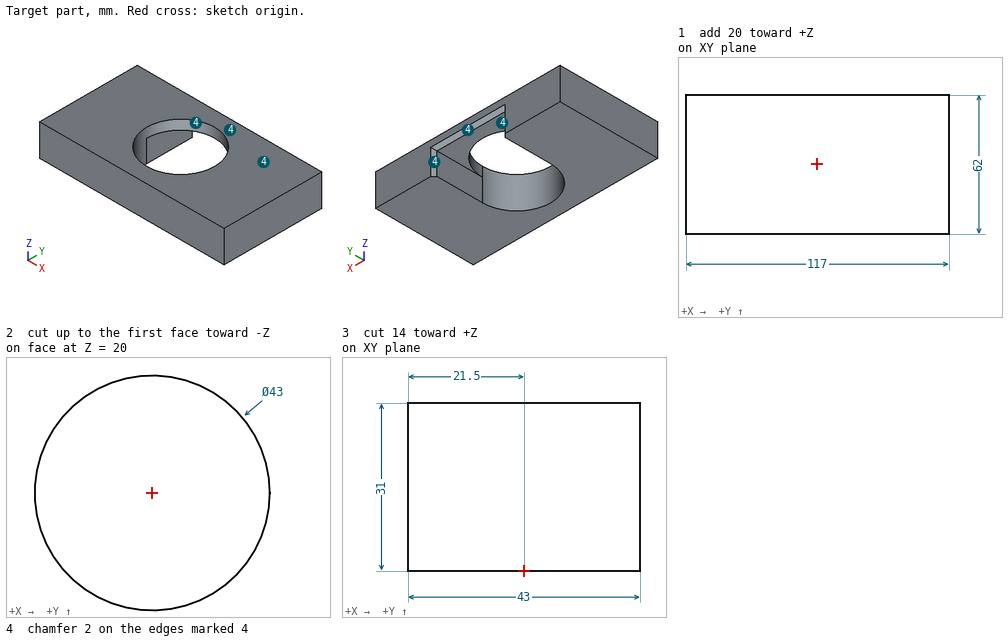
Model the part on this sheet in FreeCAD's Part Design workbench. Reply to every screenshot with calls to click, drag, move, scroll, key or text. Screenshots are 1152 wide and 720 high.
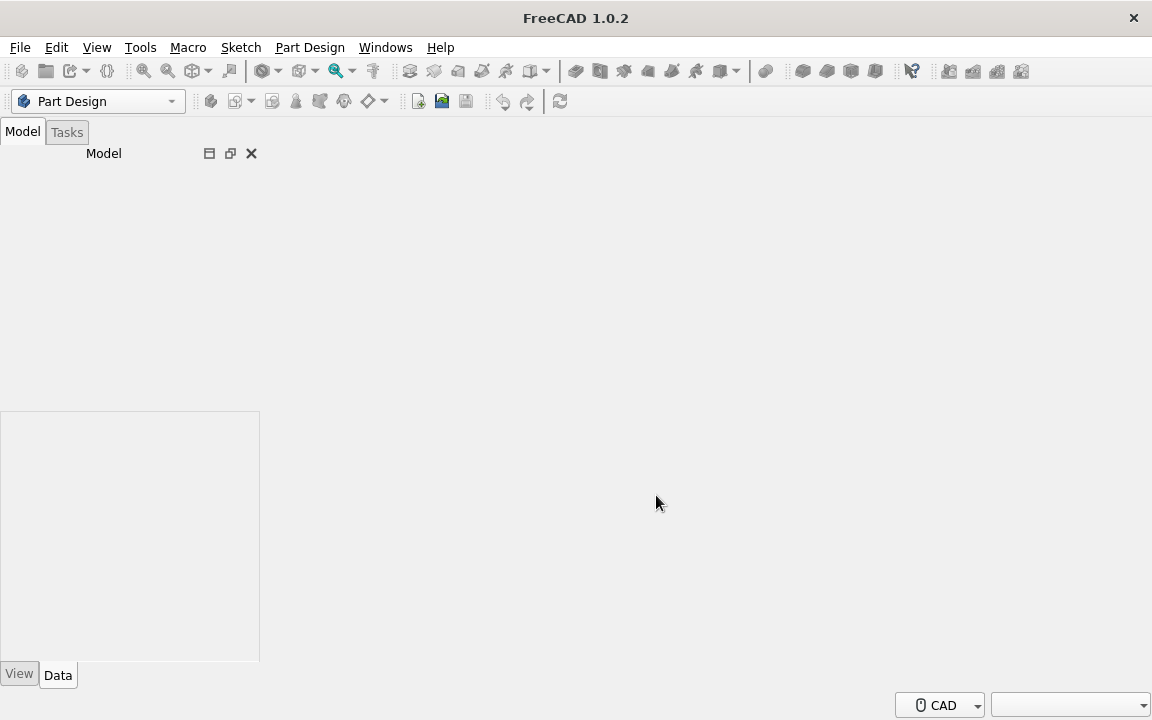
click(418, 102)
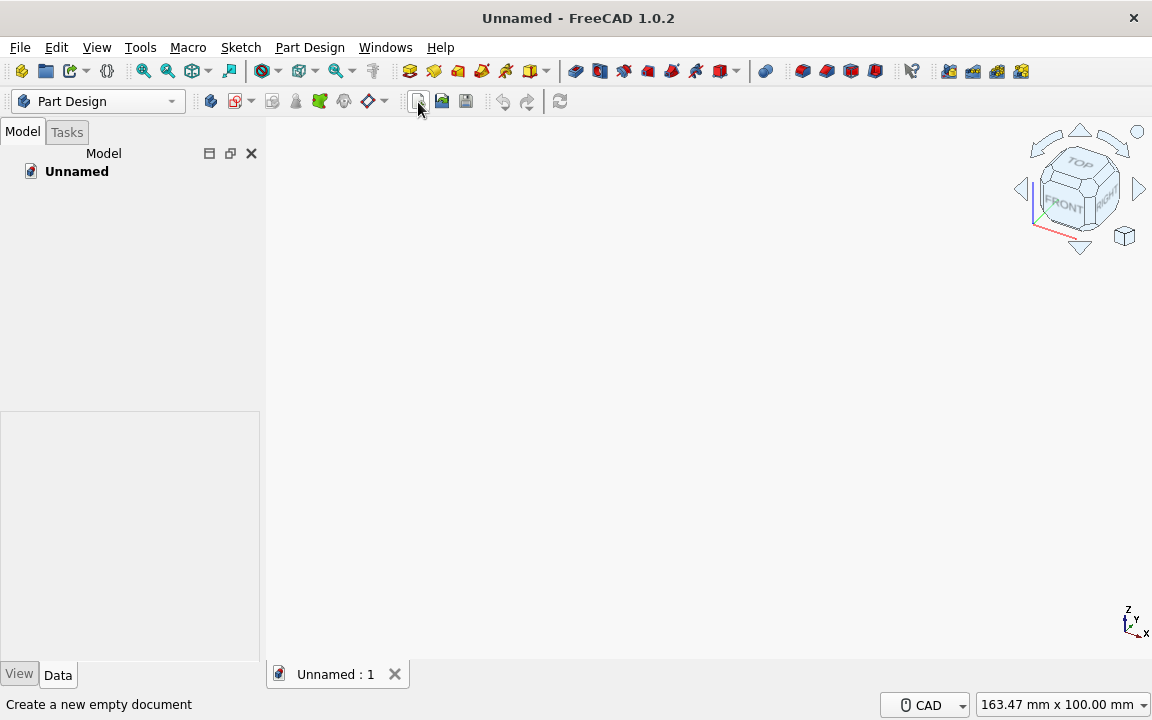
click(236, 102)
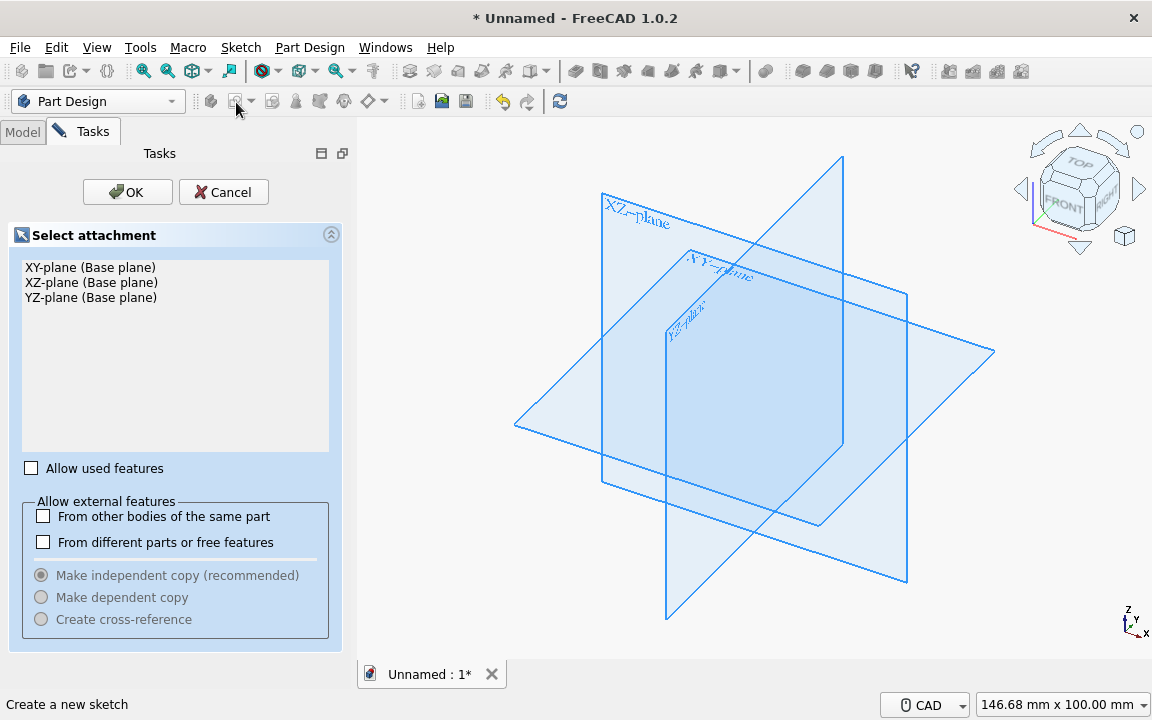
click(82, 268)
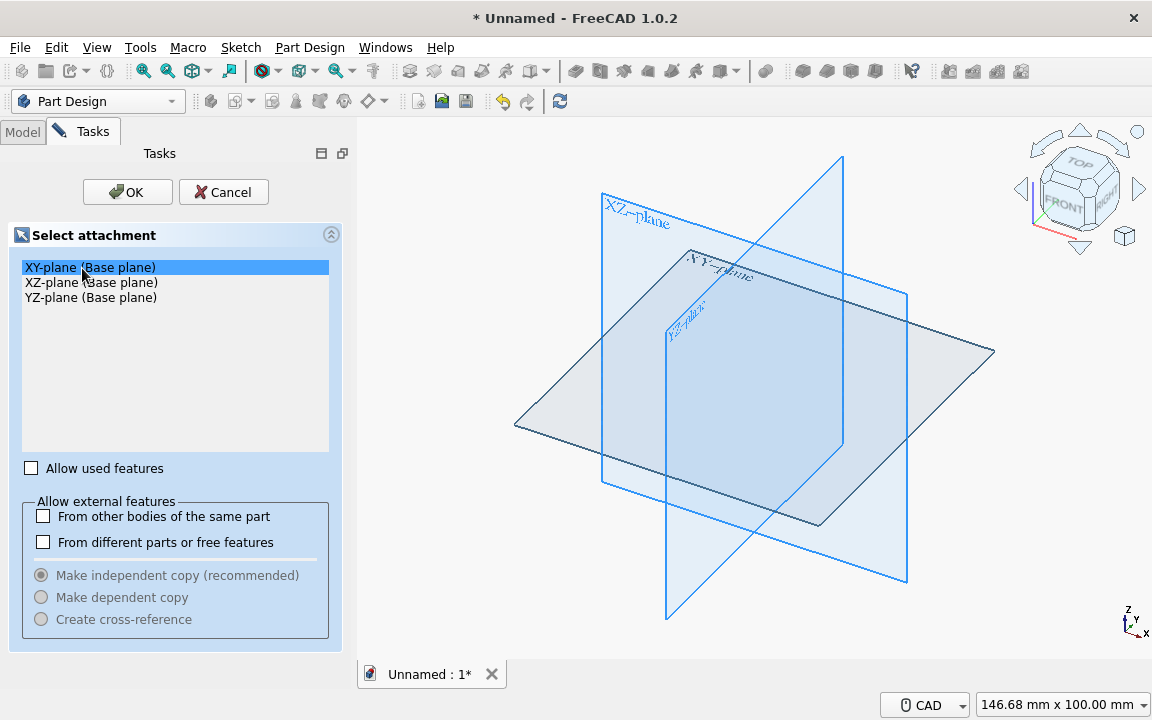
click(128, 192)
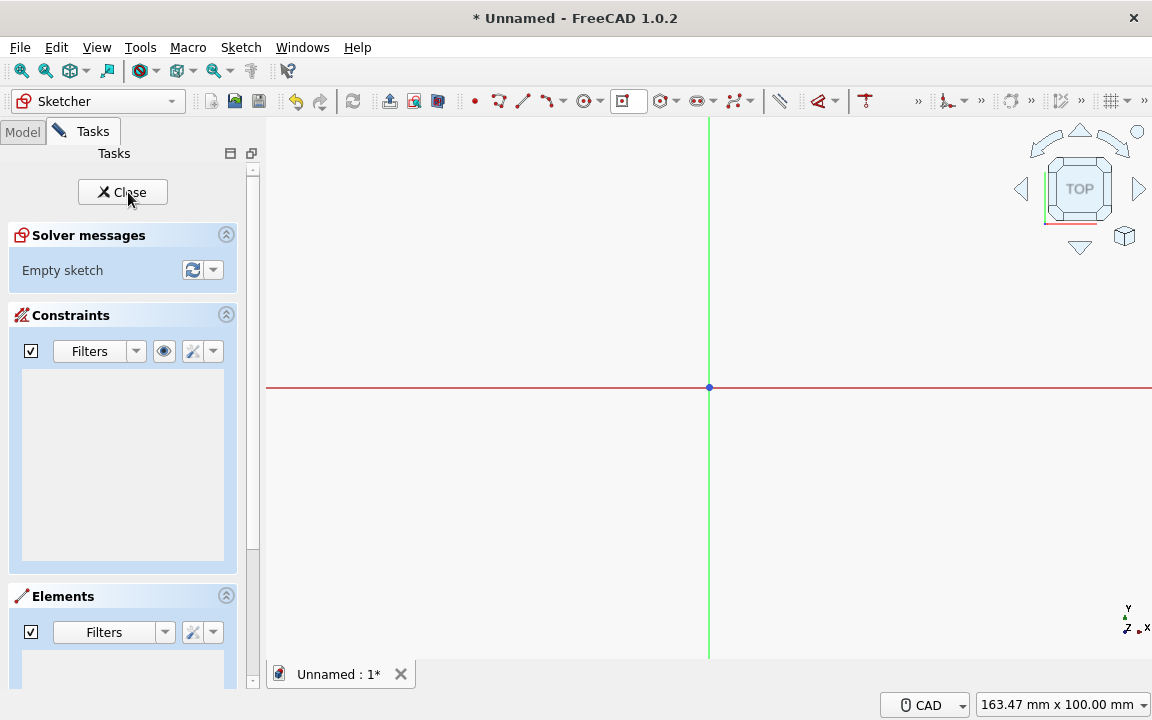
scroll(331, 388, down, 1)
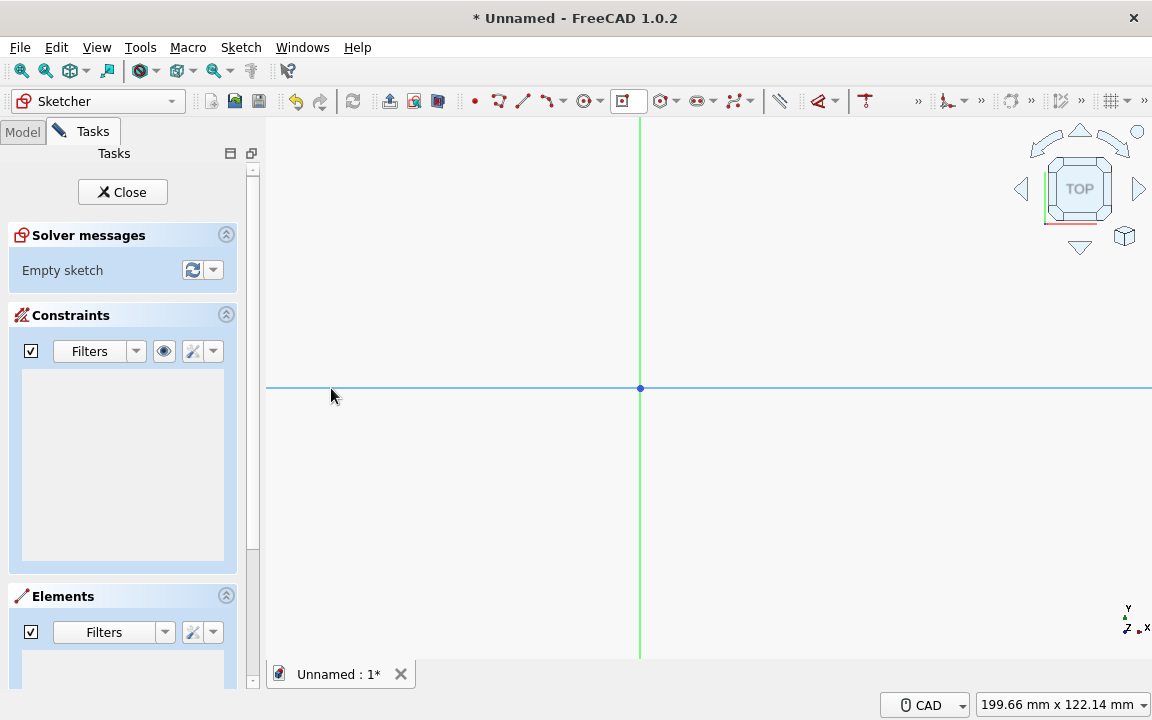
key(g)
key(v)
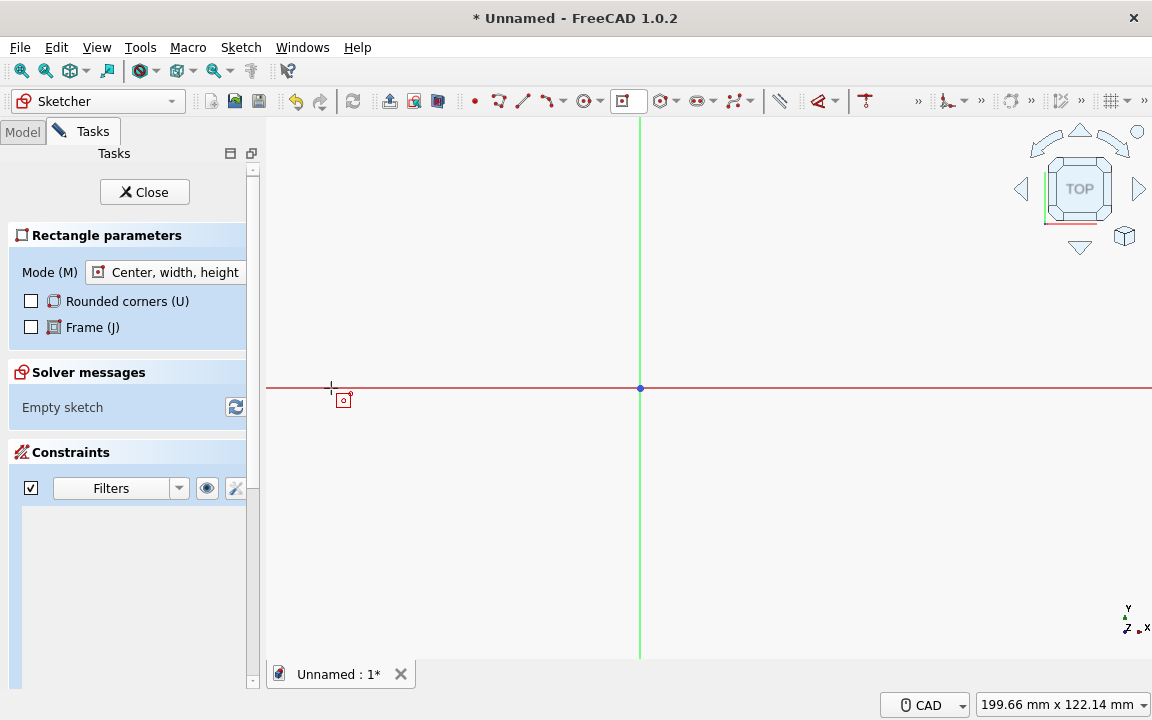
click(640, 388)
click(900, 251)
key(Escape)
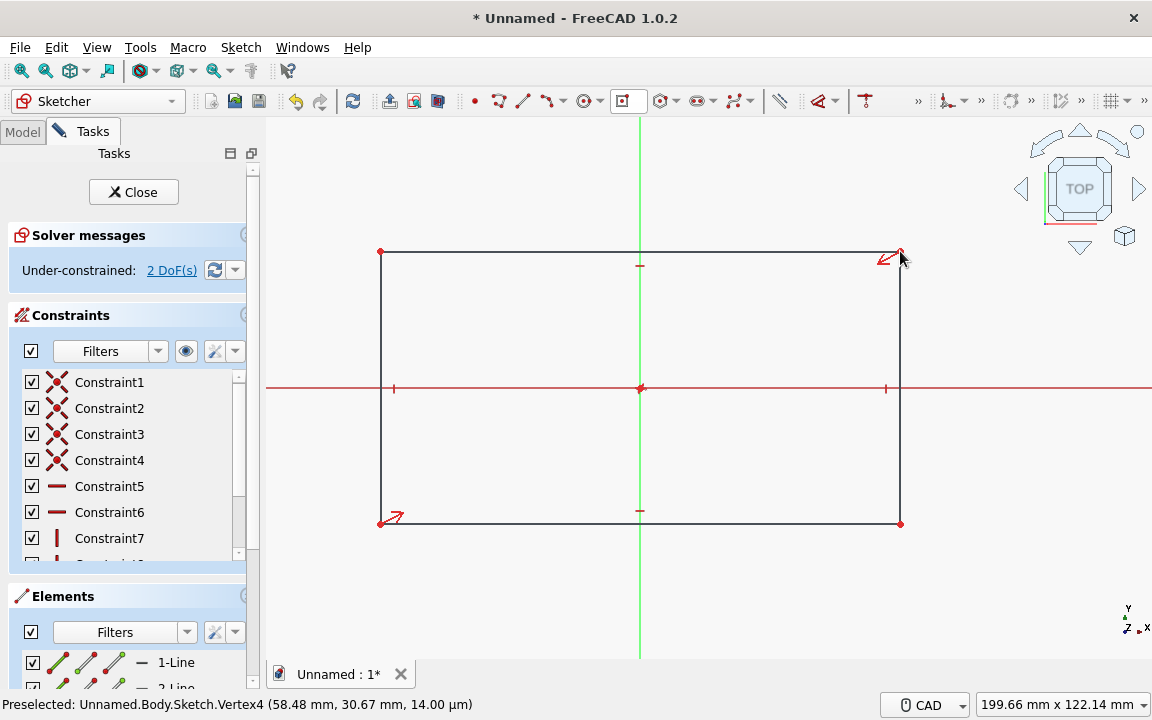
key(d)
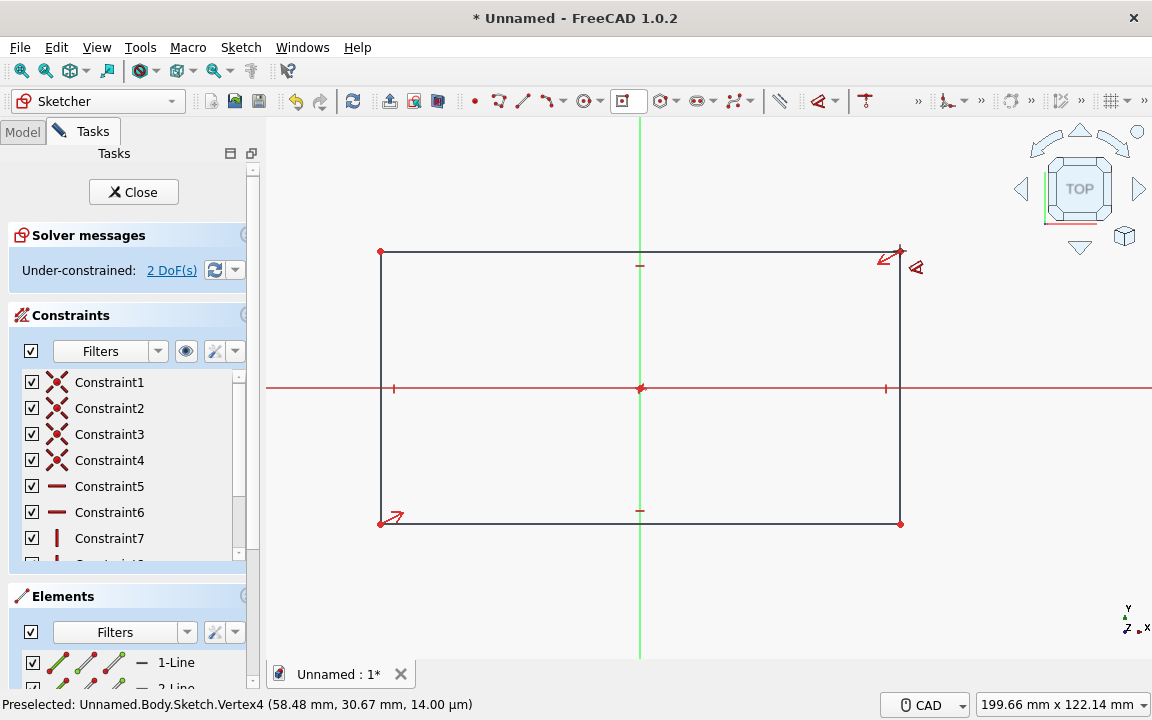
click(900, 443)
click(934, 325)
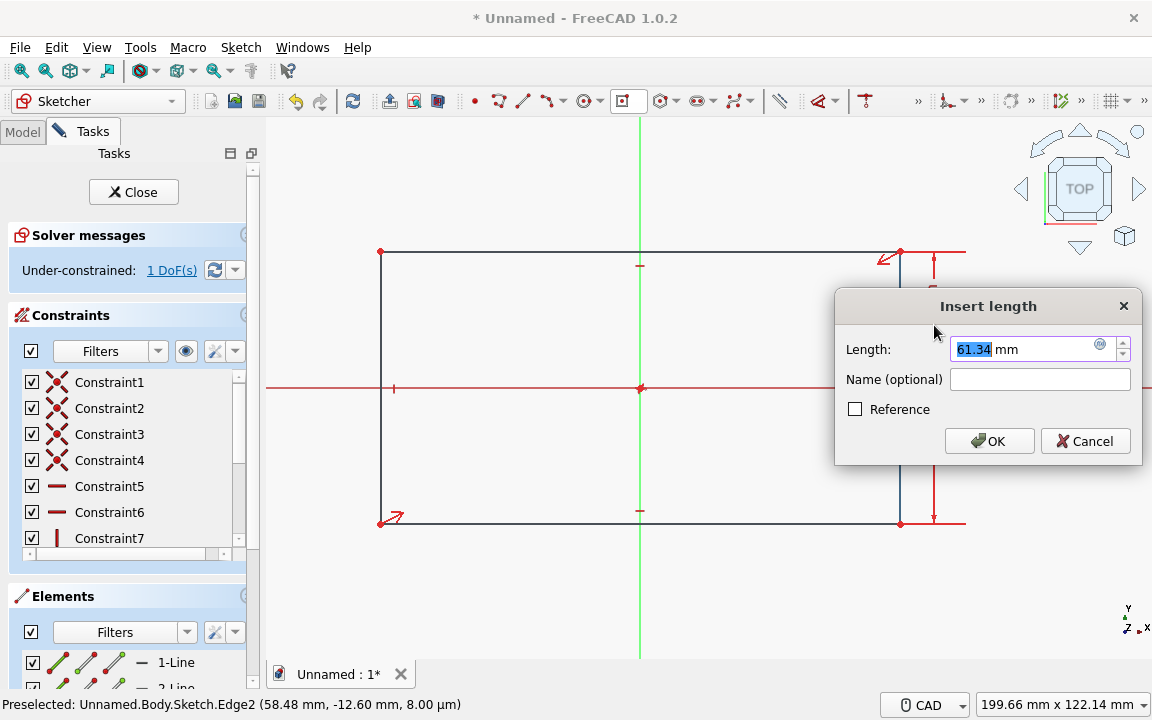
text(62)
key(Return)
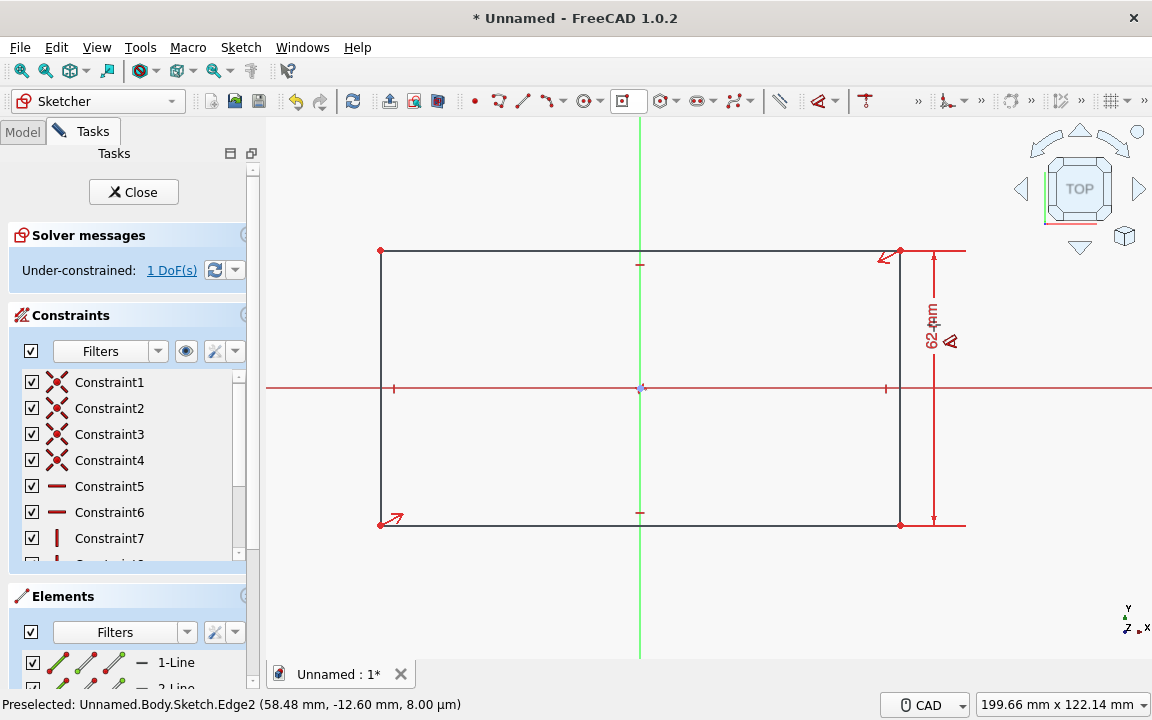
click(537, 526)
click(521, 560)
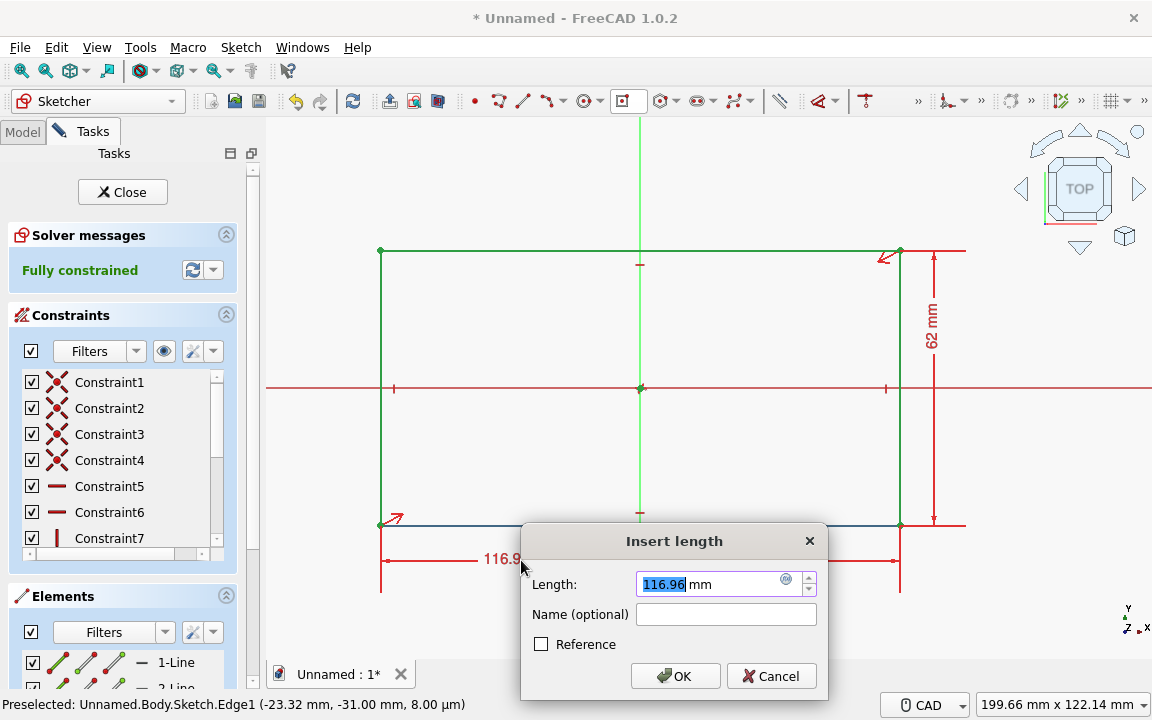
text(117)
key(Return)
key(Escape)